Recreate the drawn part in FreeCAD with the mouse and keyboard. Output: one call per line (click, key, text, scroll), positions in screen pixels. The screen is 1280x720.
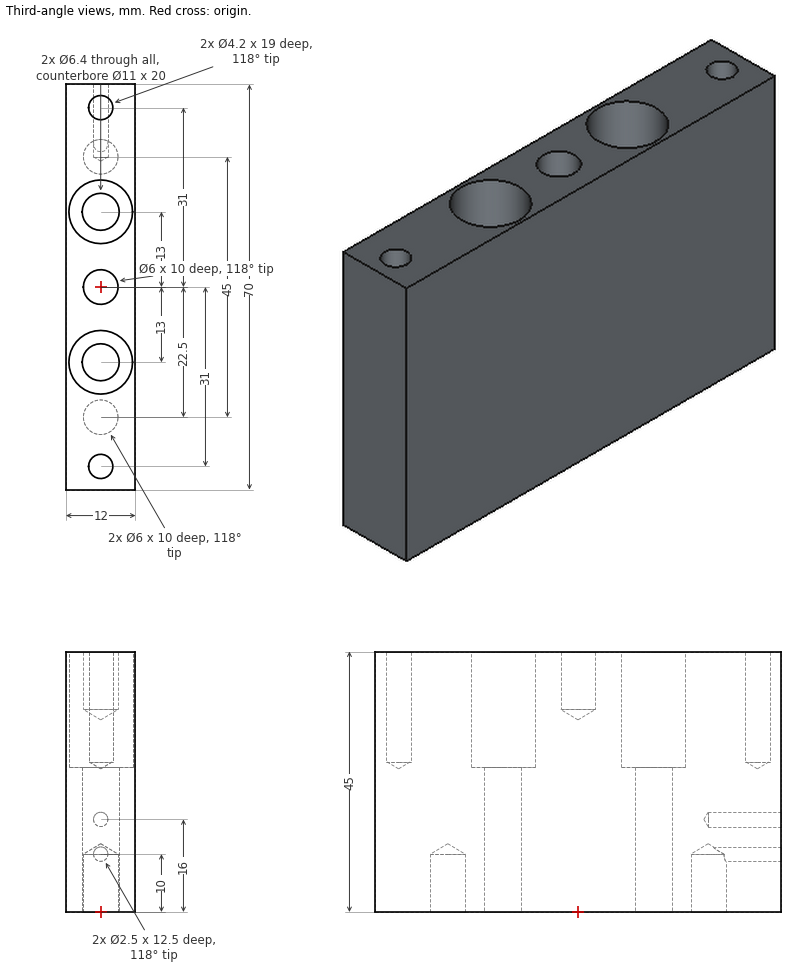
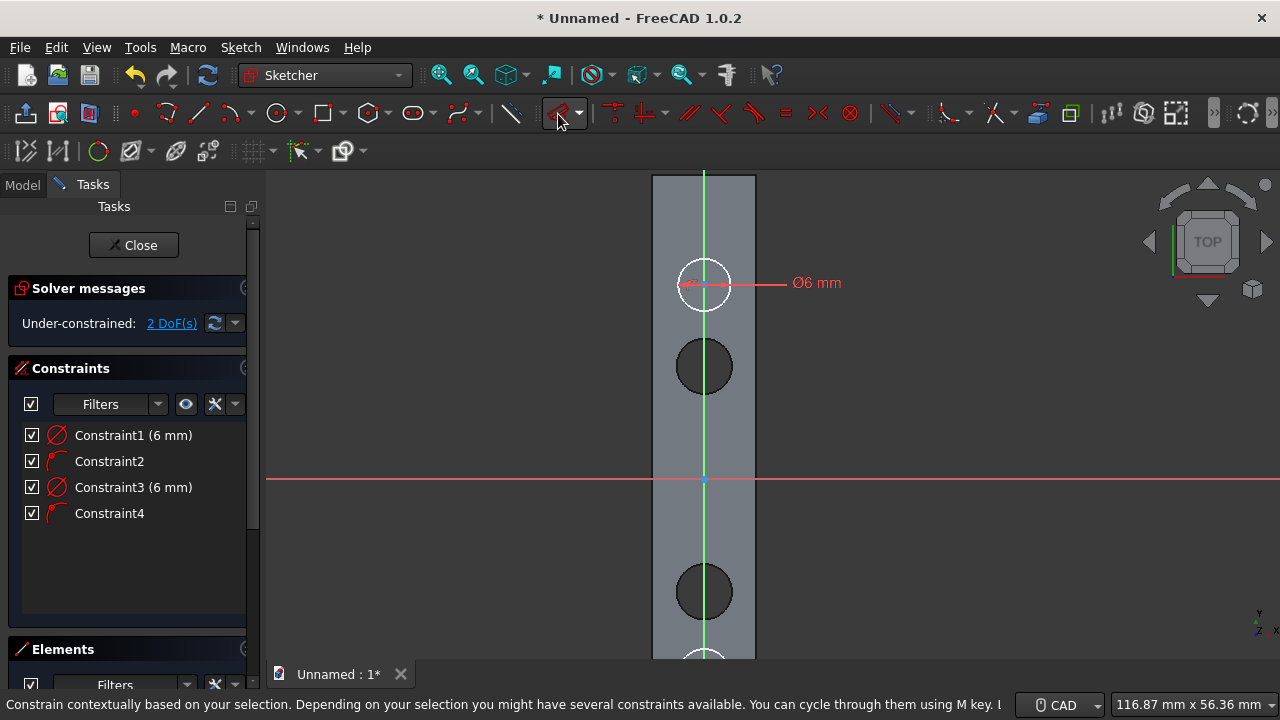
scroll(705, 283, down, 2)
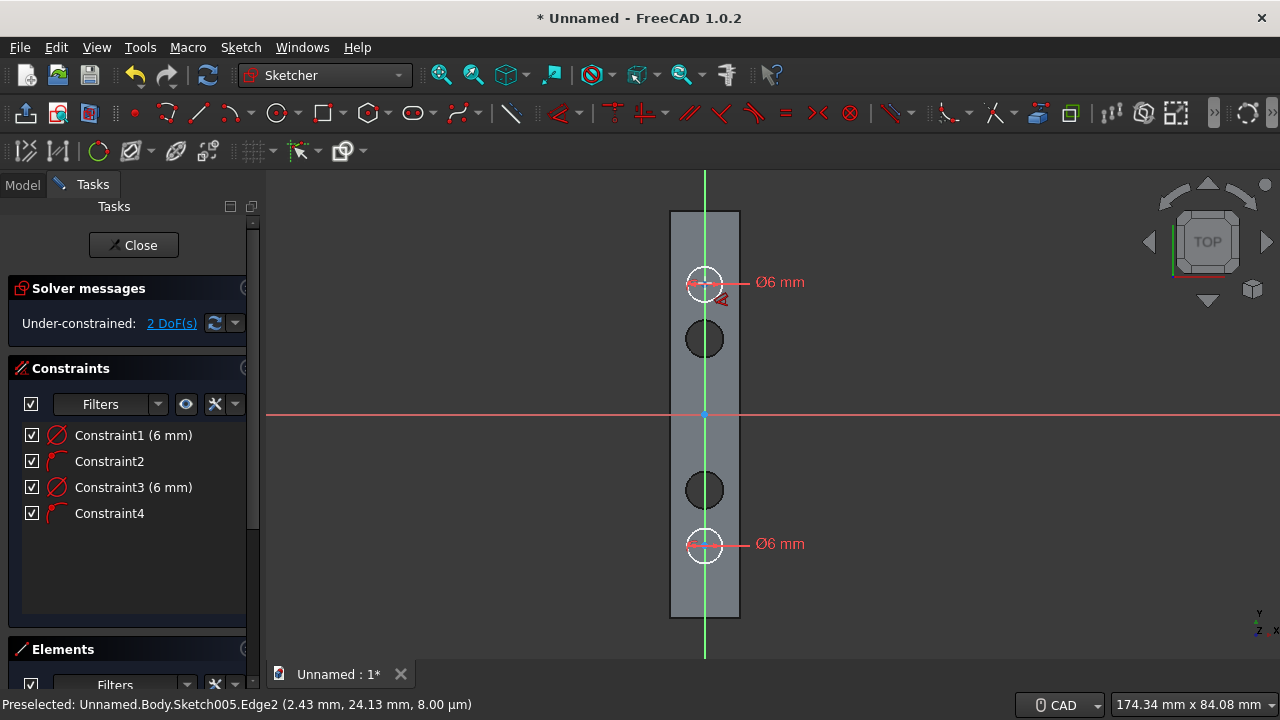
click(705, 546)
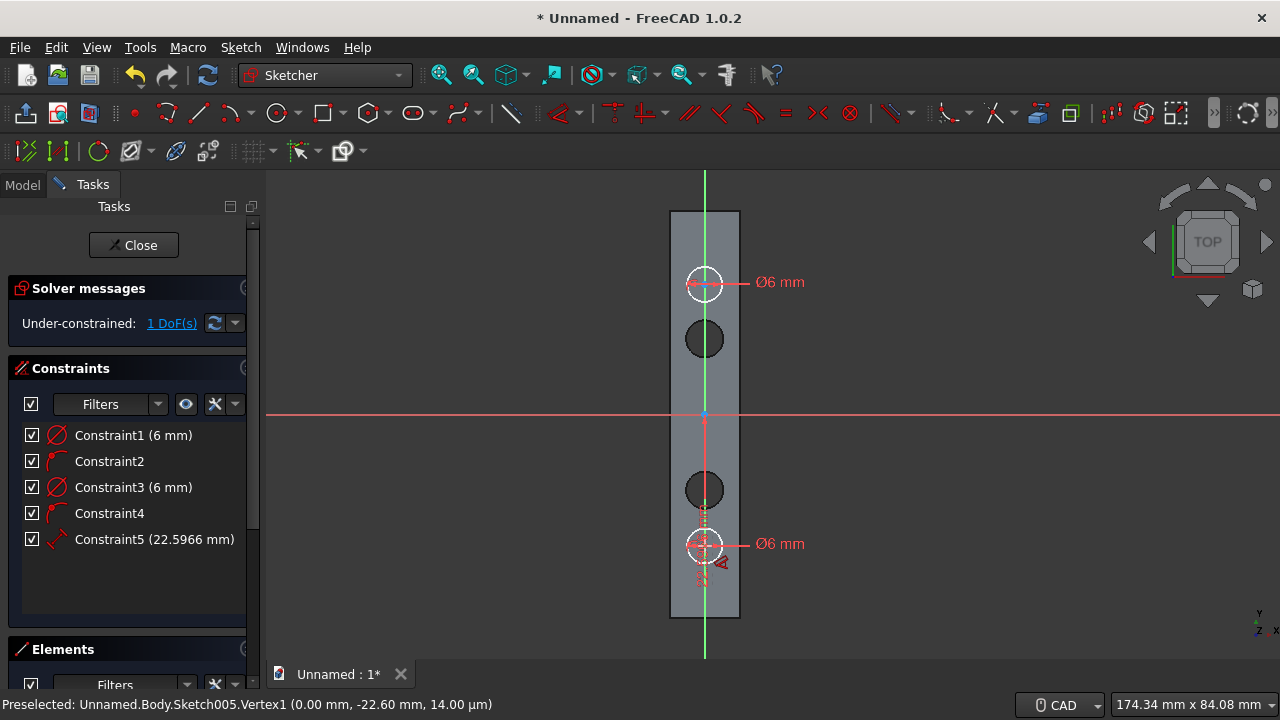
click(705, 284)
click(739, 355)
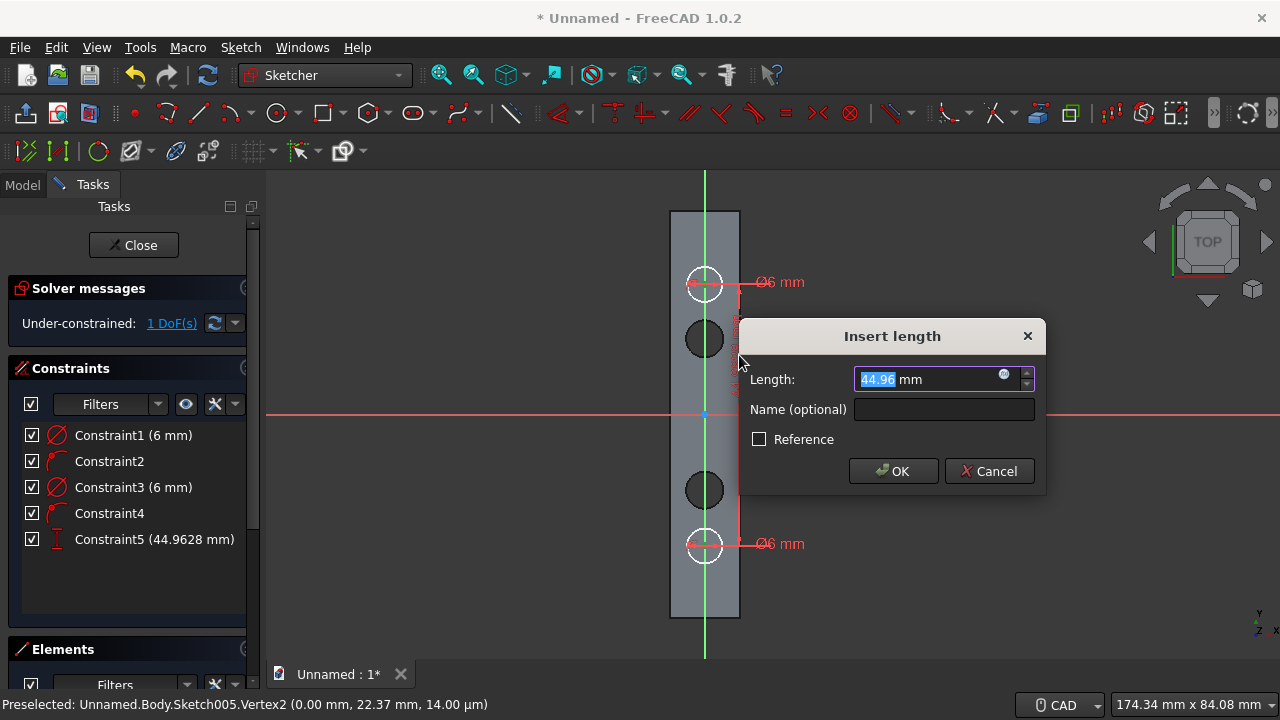
text(45)
key(Return)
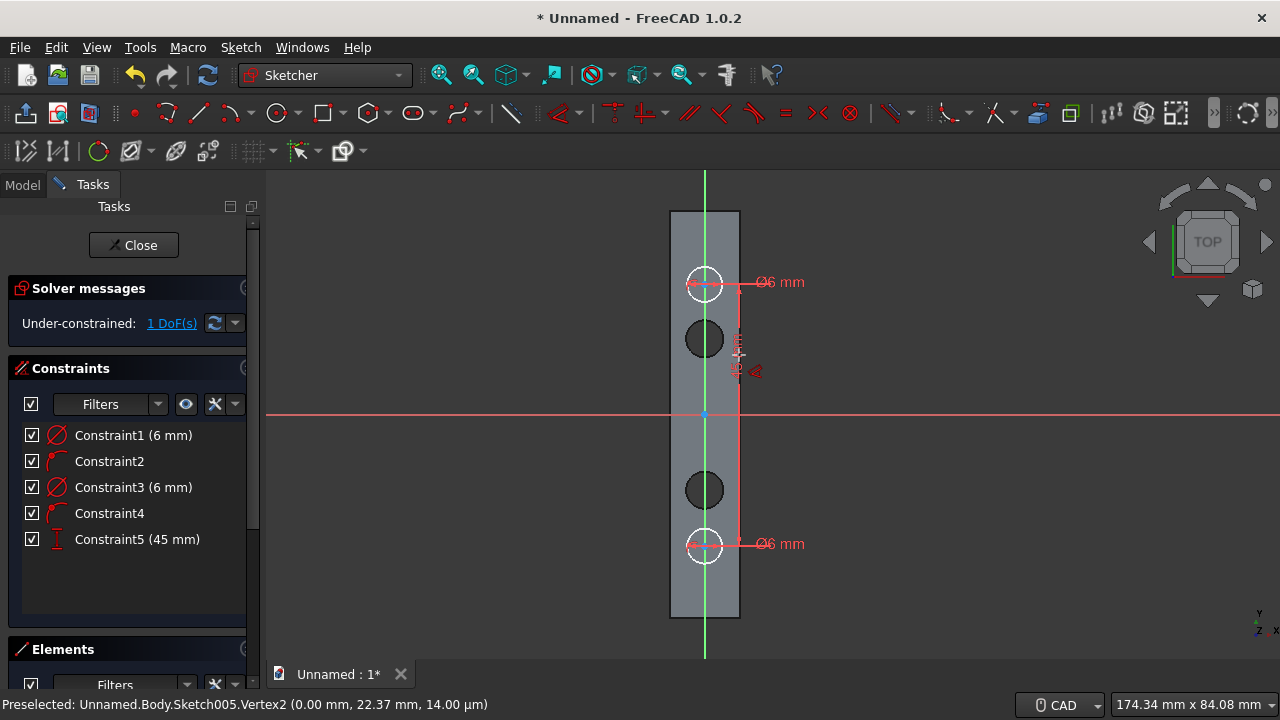
click(705, 546)
click(739, 480)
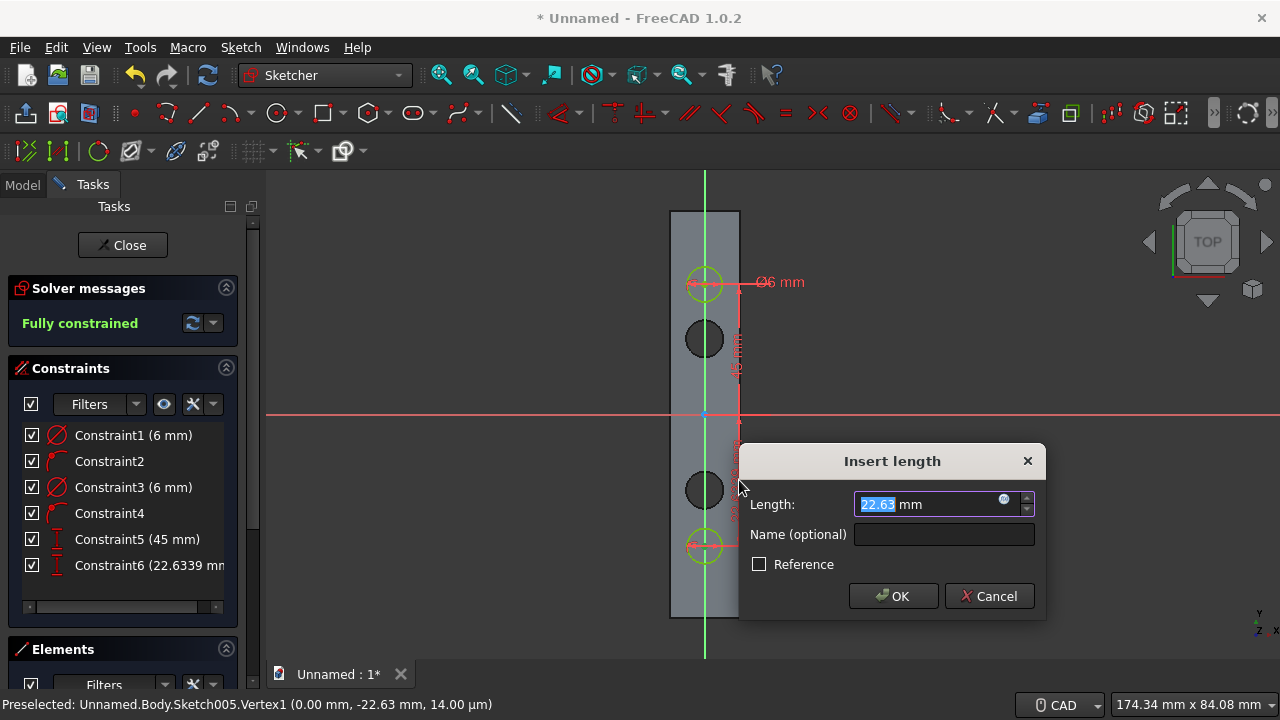
text(22.5)
key(Return)
key(Escape)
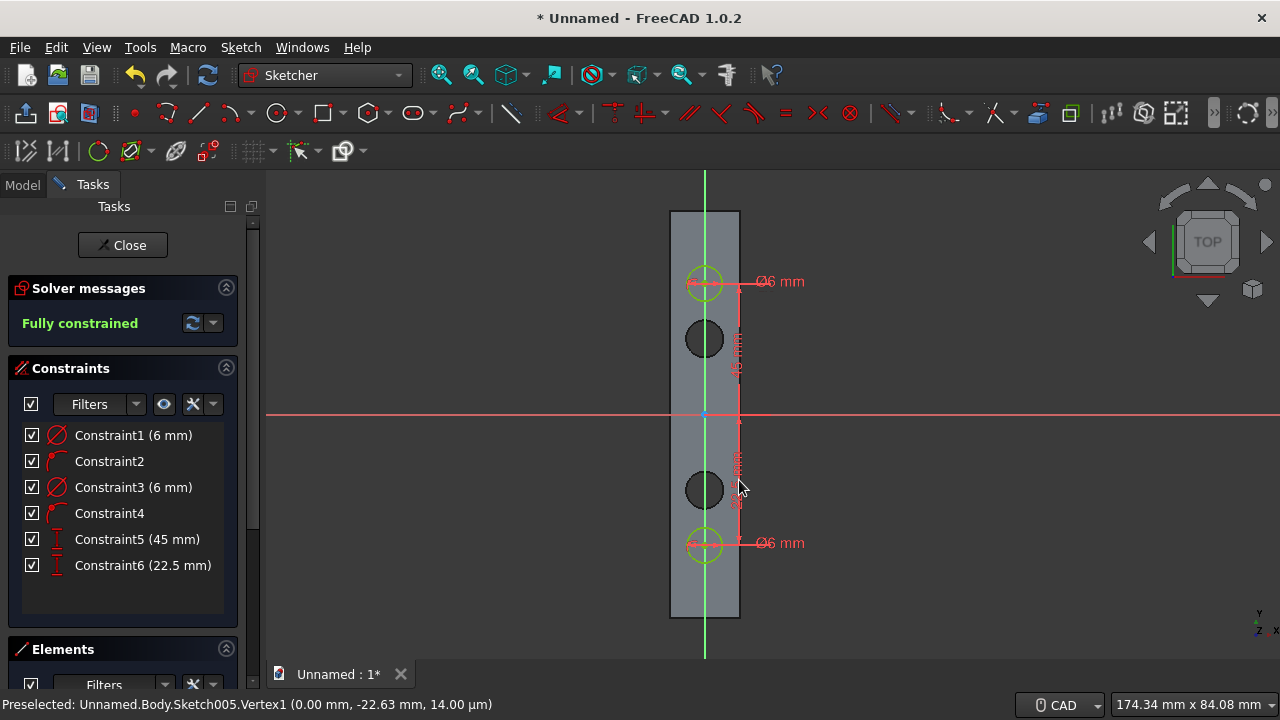
click(123, 245)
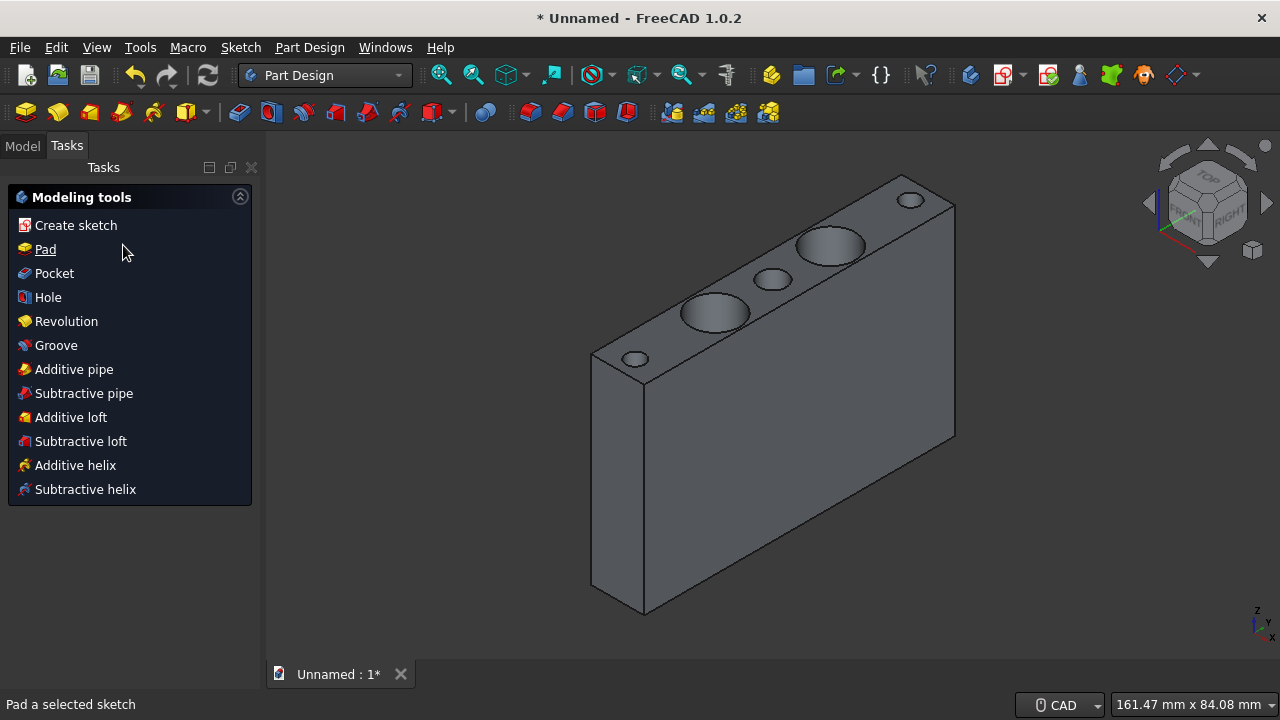
click(272, 112)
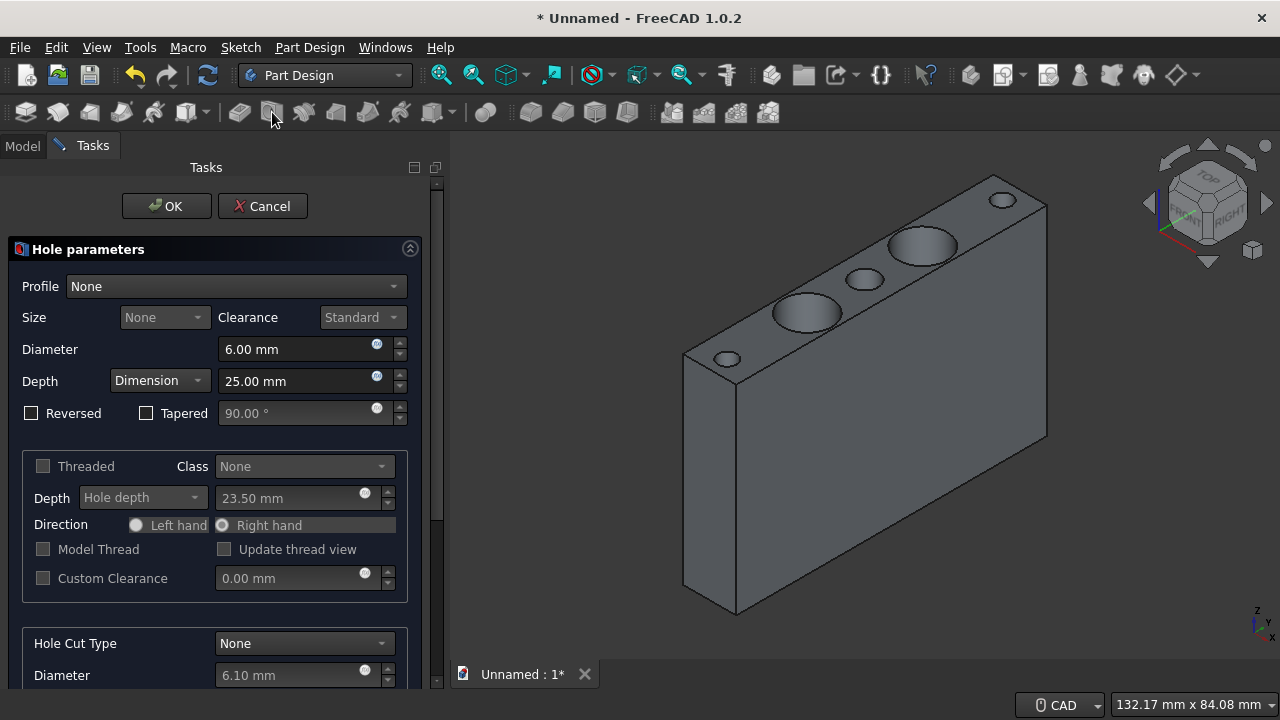
triple_click(305, 349)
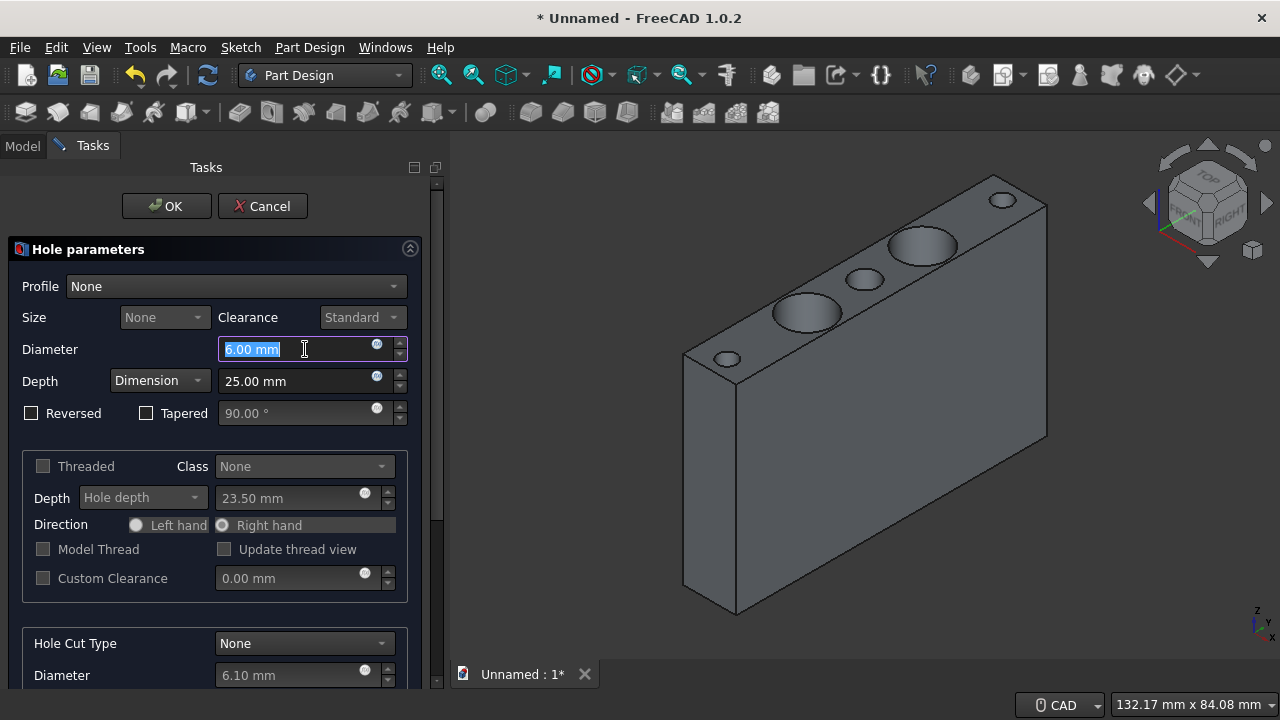
text(6)
key(Tab)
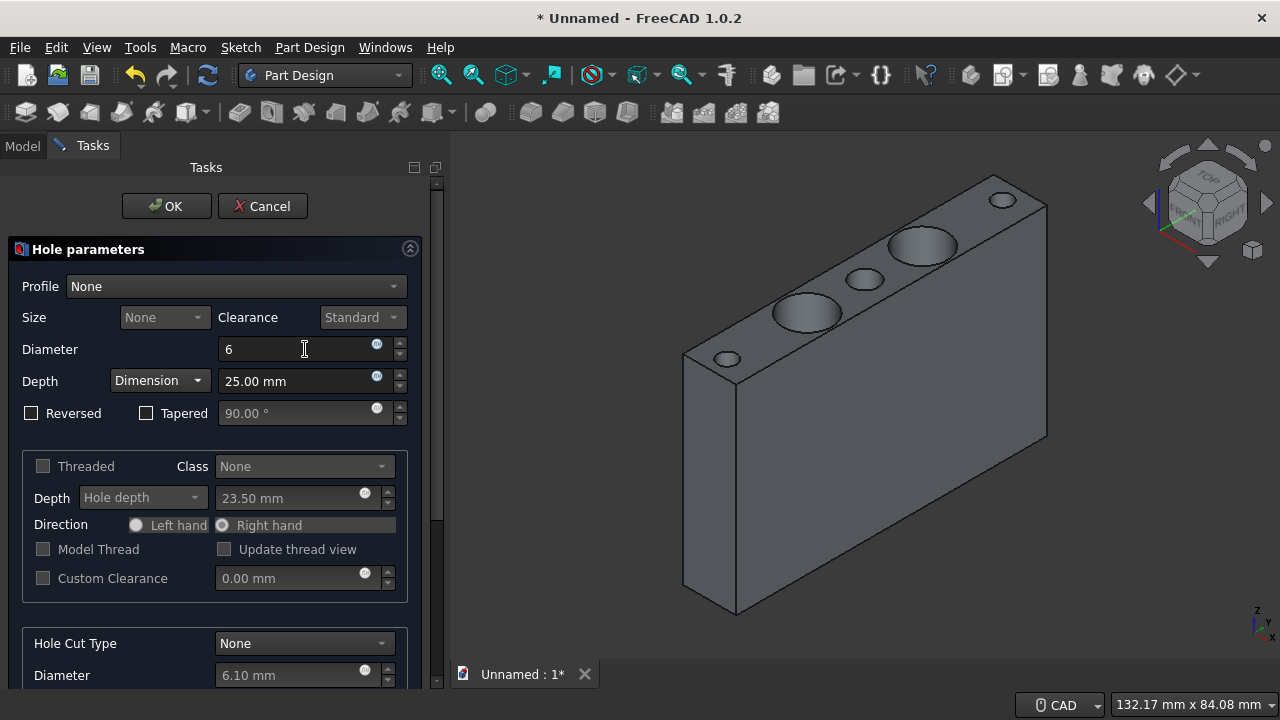
triple_click(305, 381)